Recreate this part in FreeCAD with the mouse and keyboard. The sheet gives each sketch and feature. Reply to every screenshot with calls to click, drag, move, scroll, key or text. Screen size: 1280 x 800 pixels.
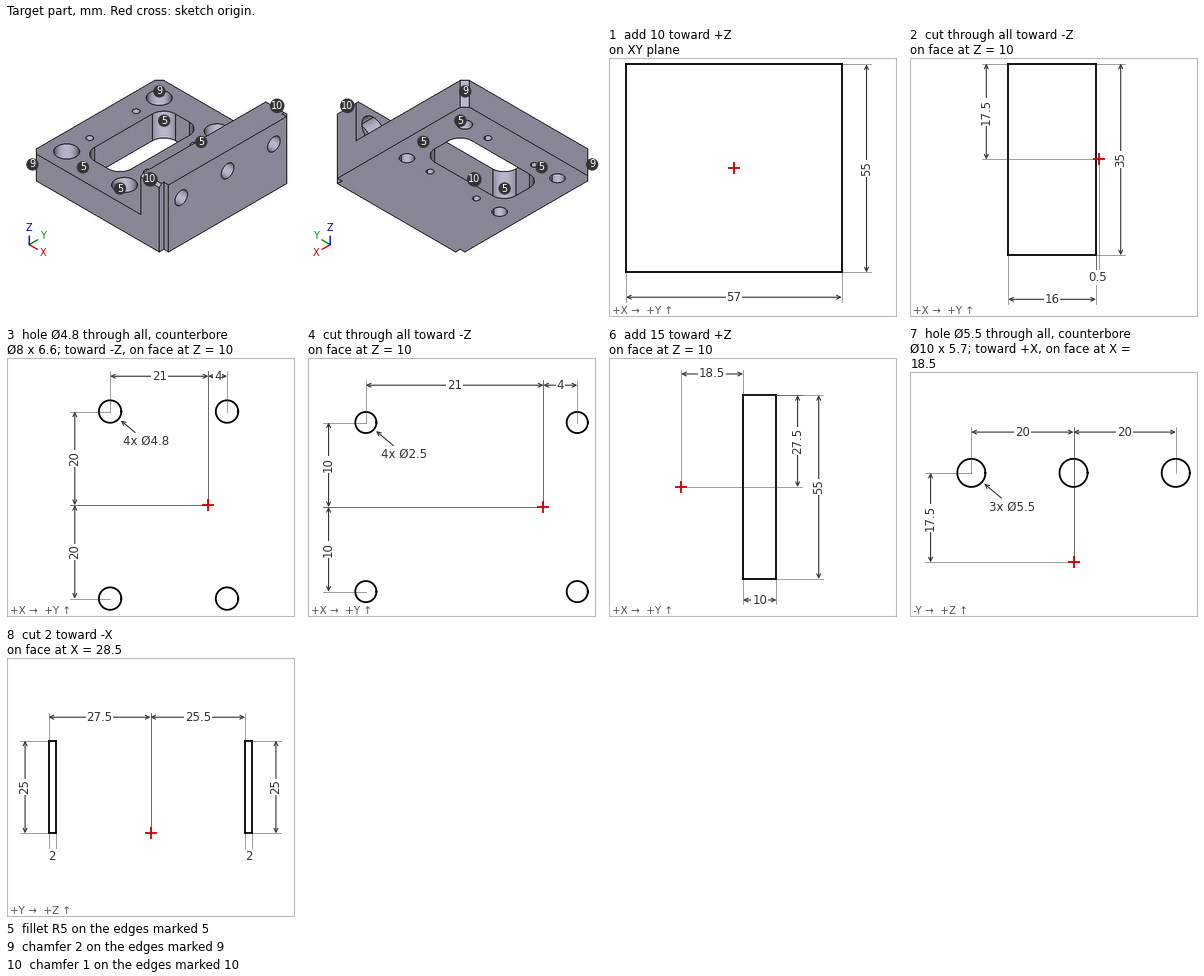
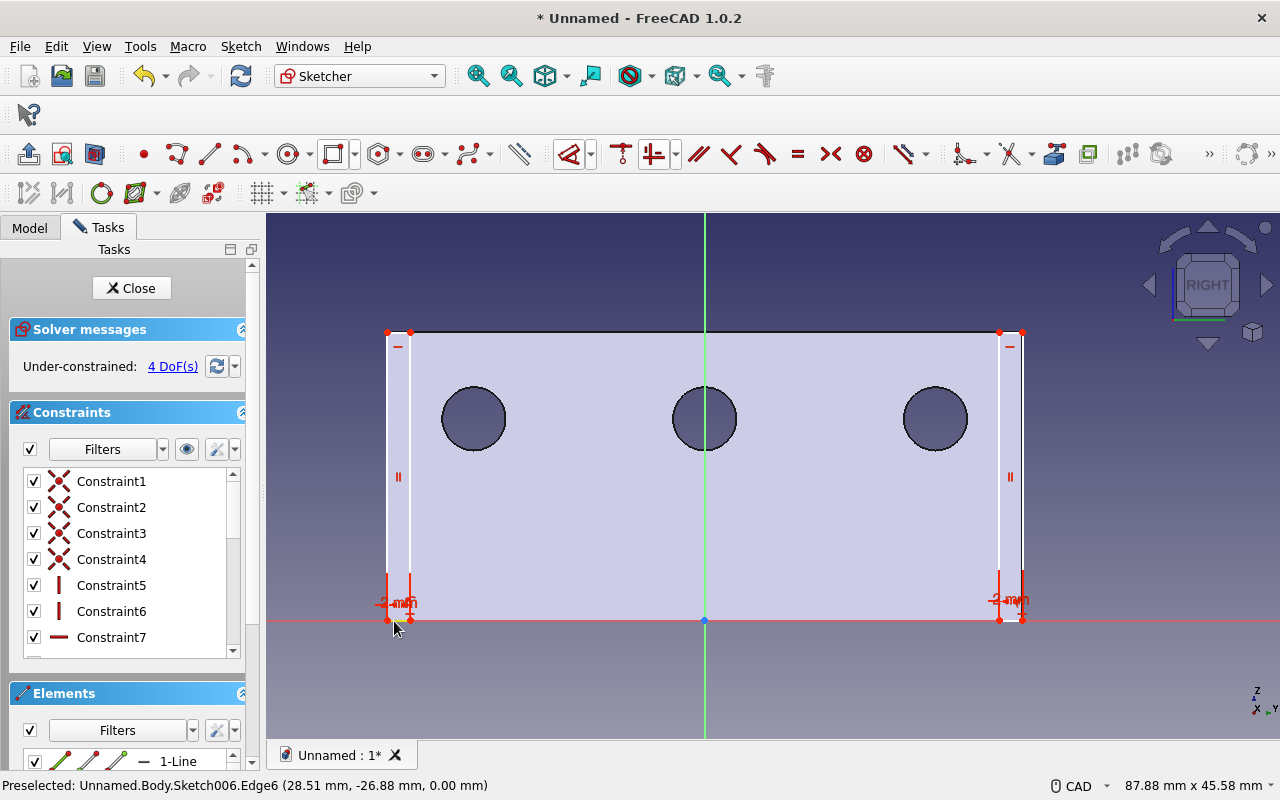
click(999, 419)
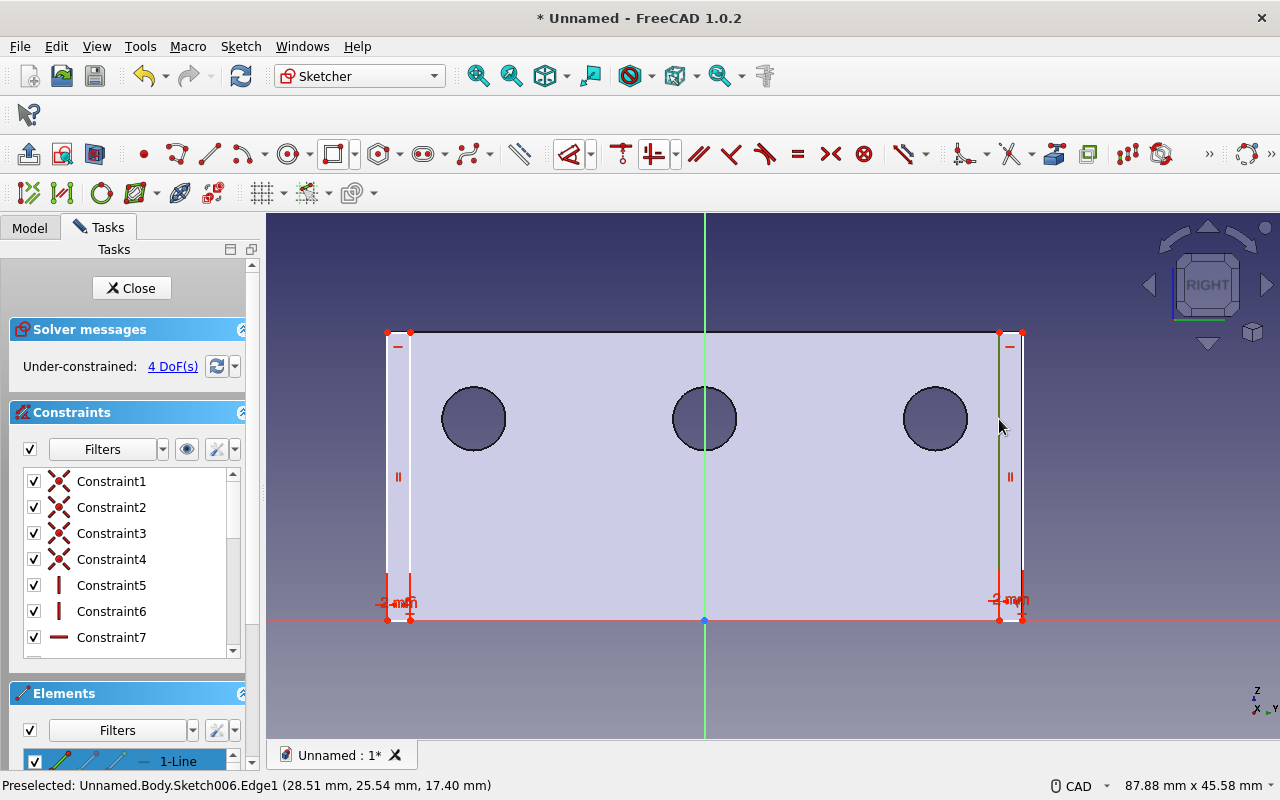
click(590, 154)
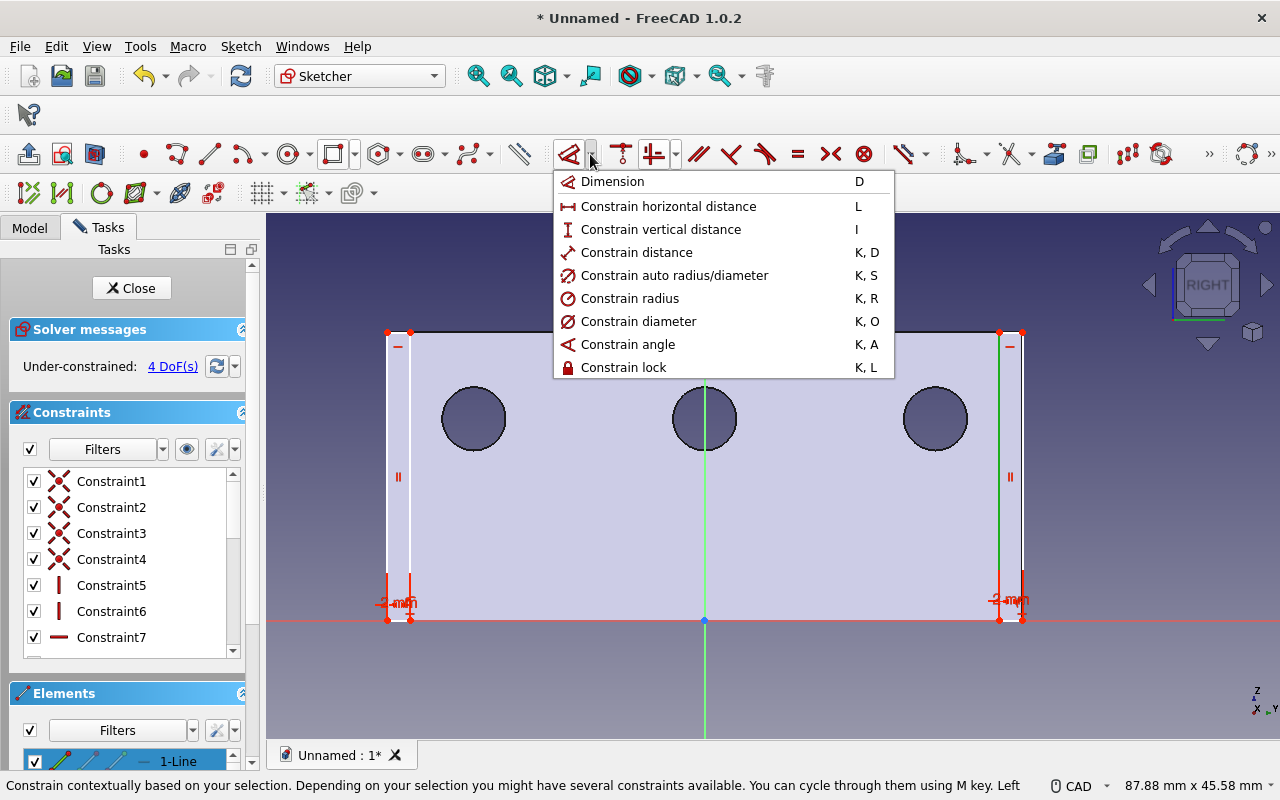
click(724, 230)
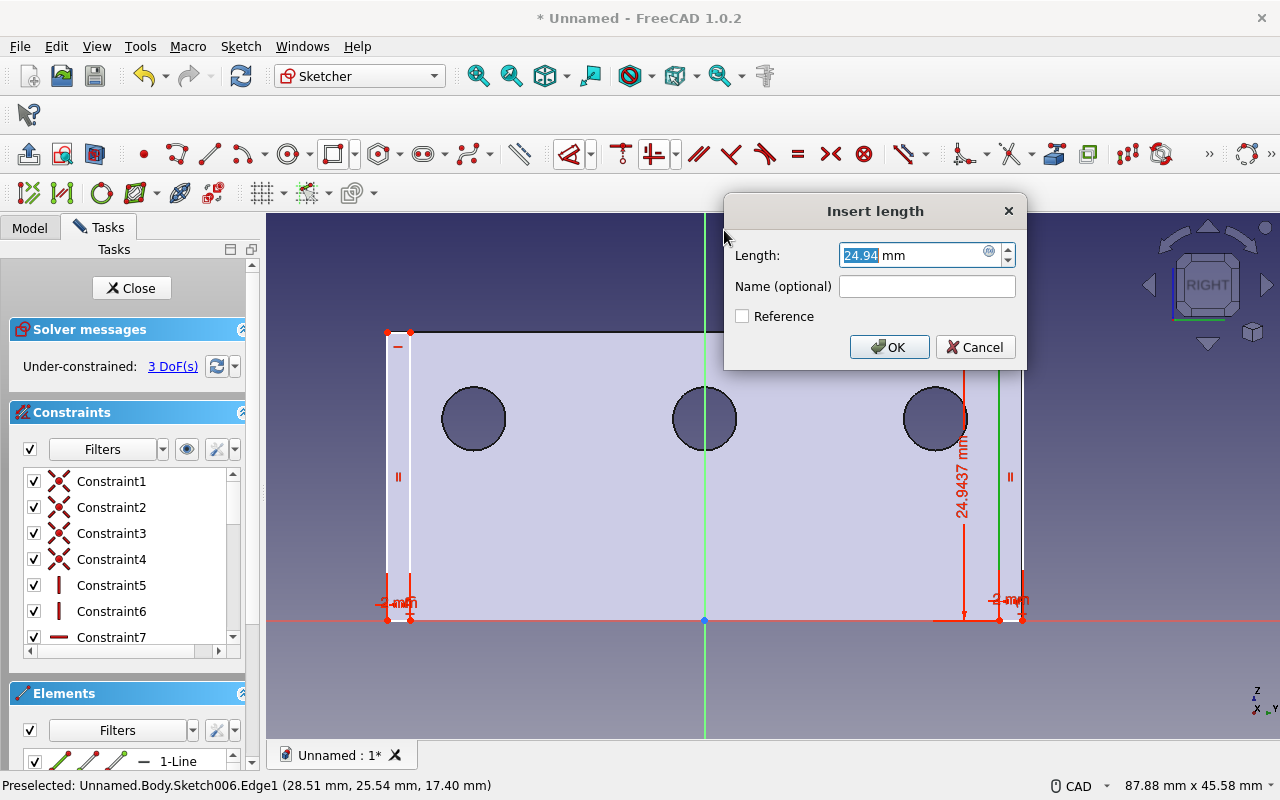
text(25)
key(Return)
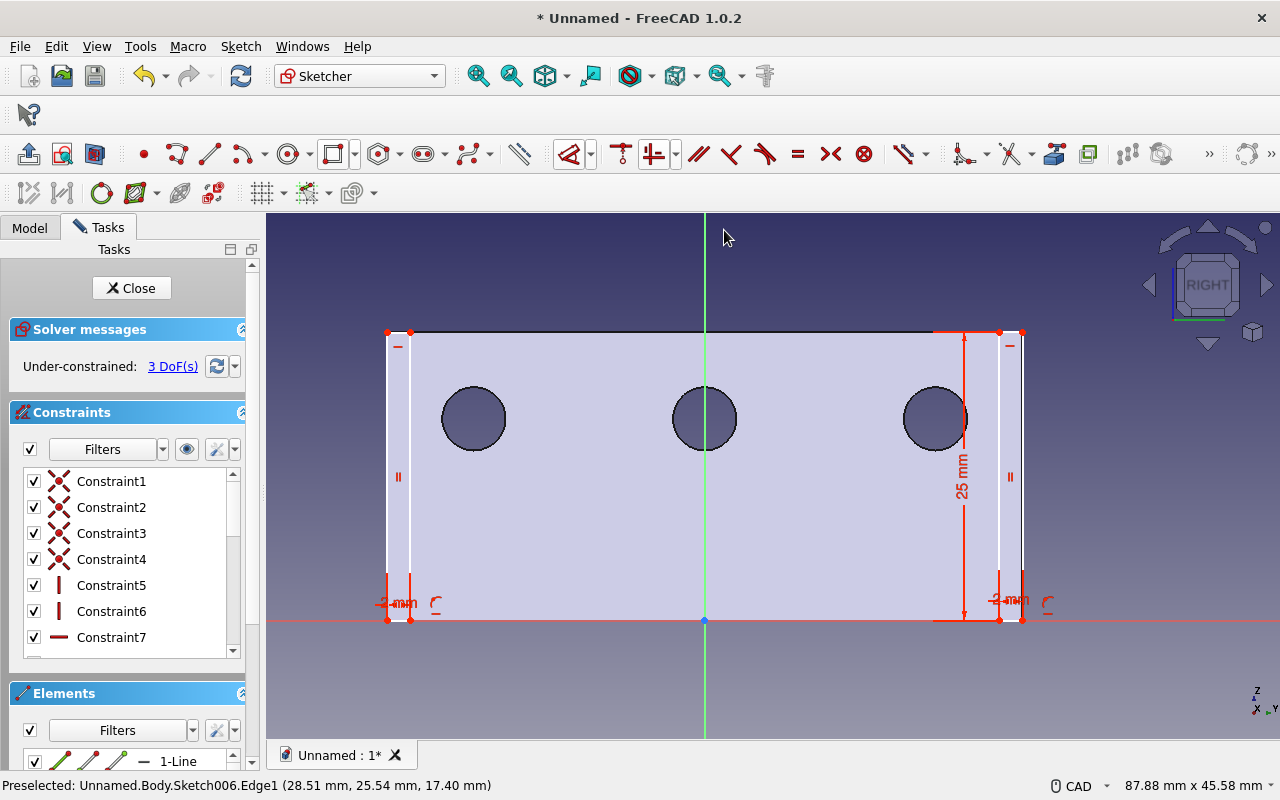
click(387, 419)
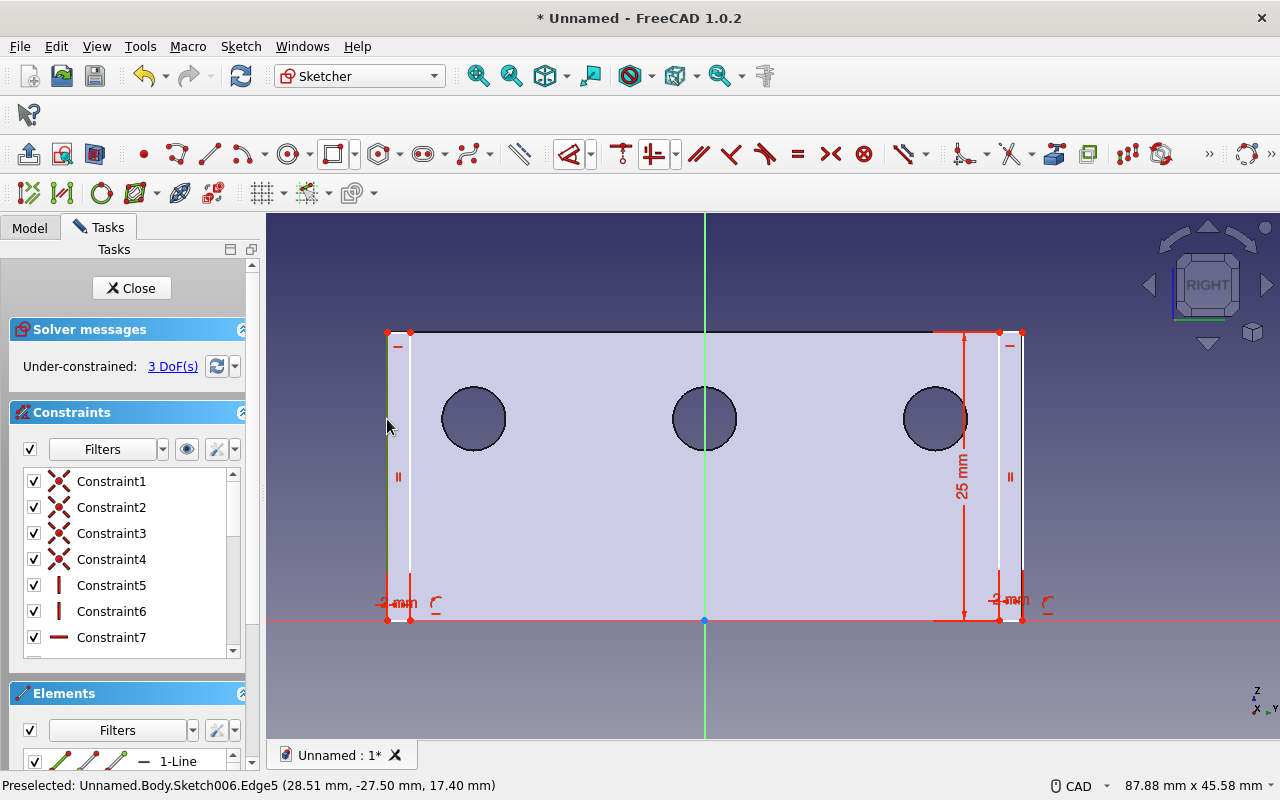
key(i)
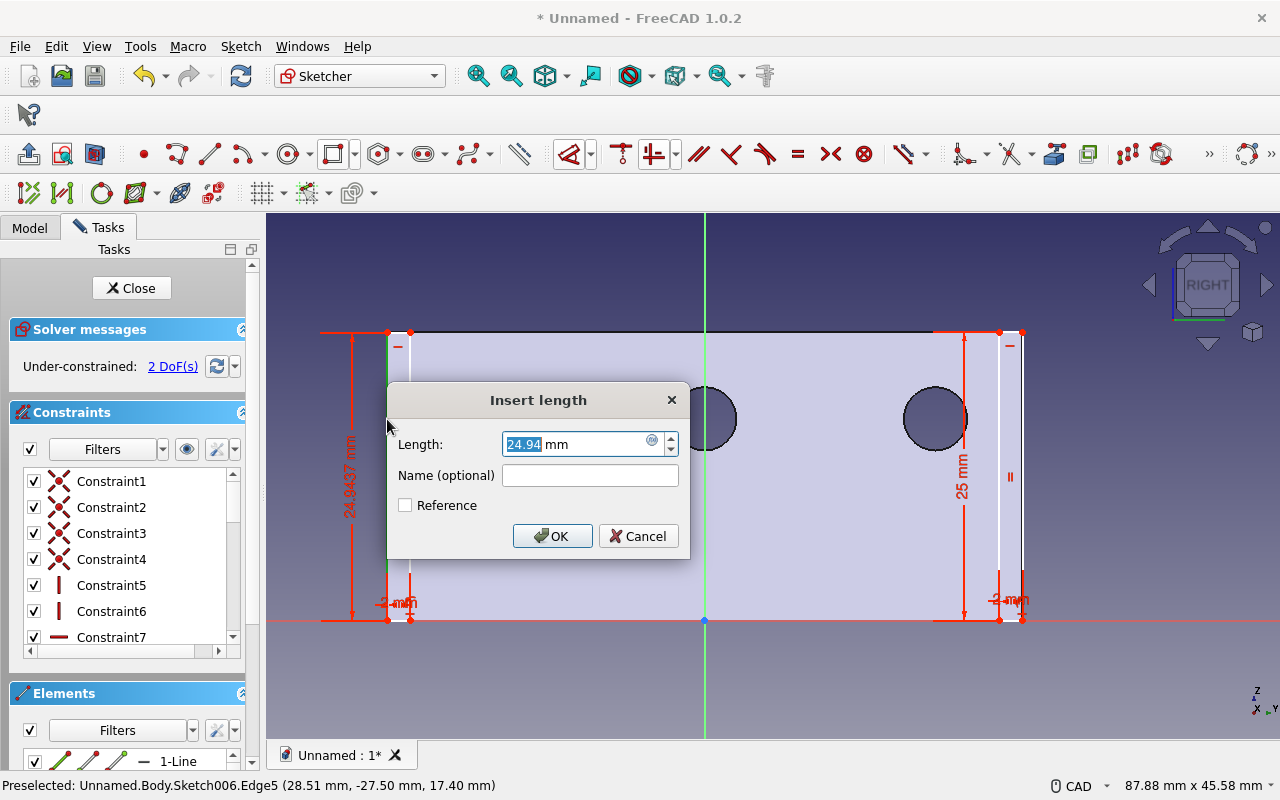
text(25)
key(Return)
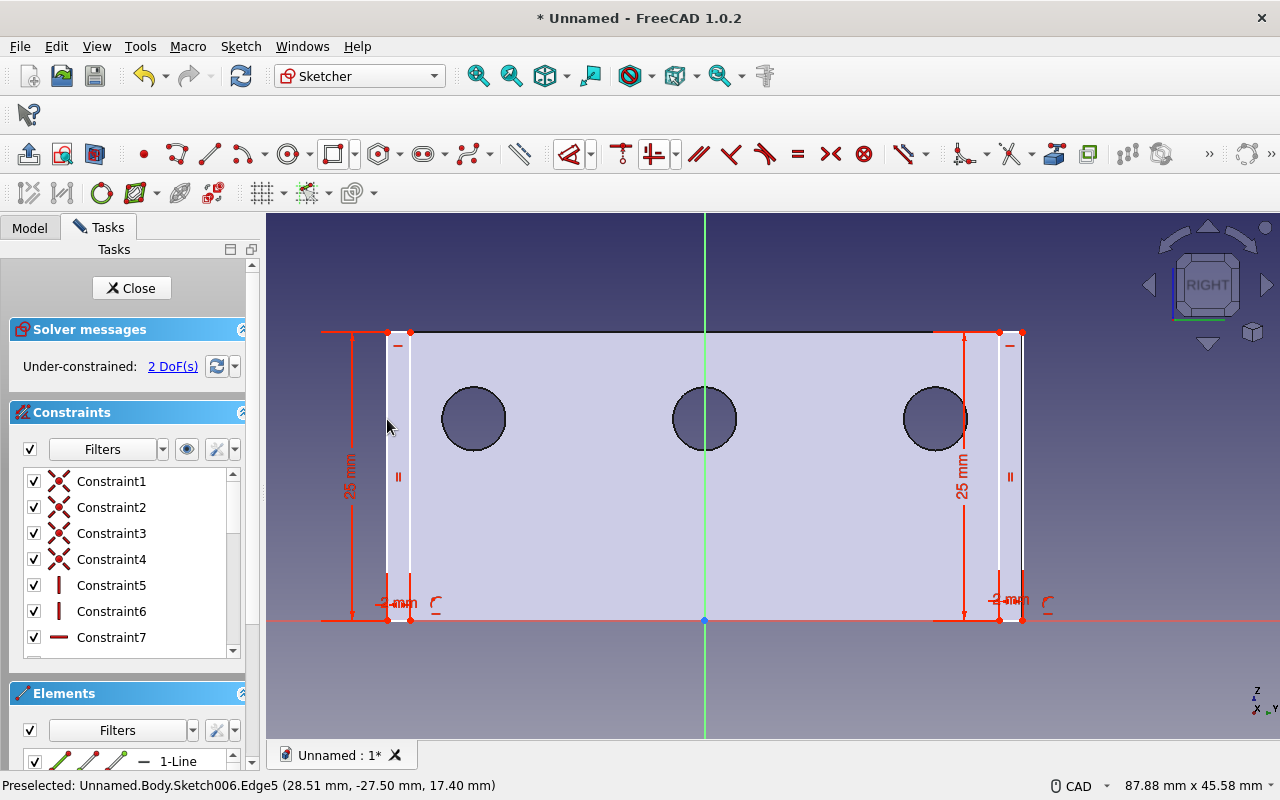
click(999, 332)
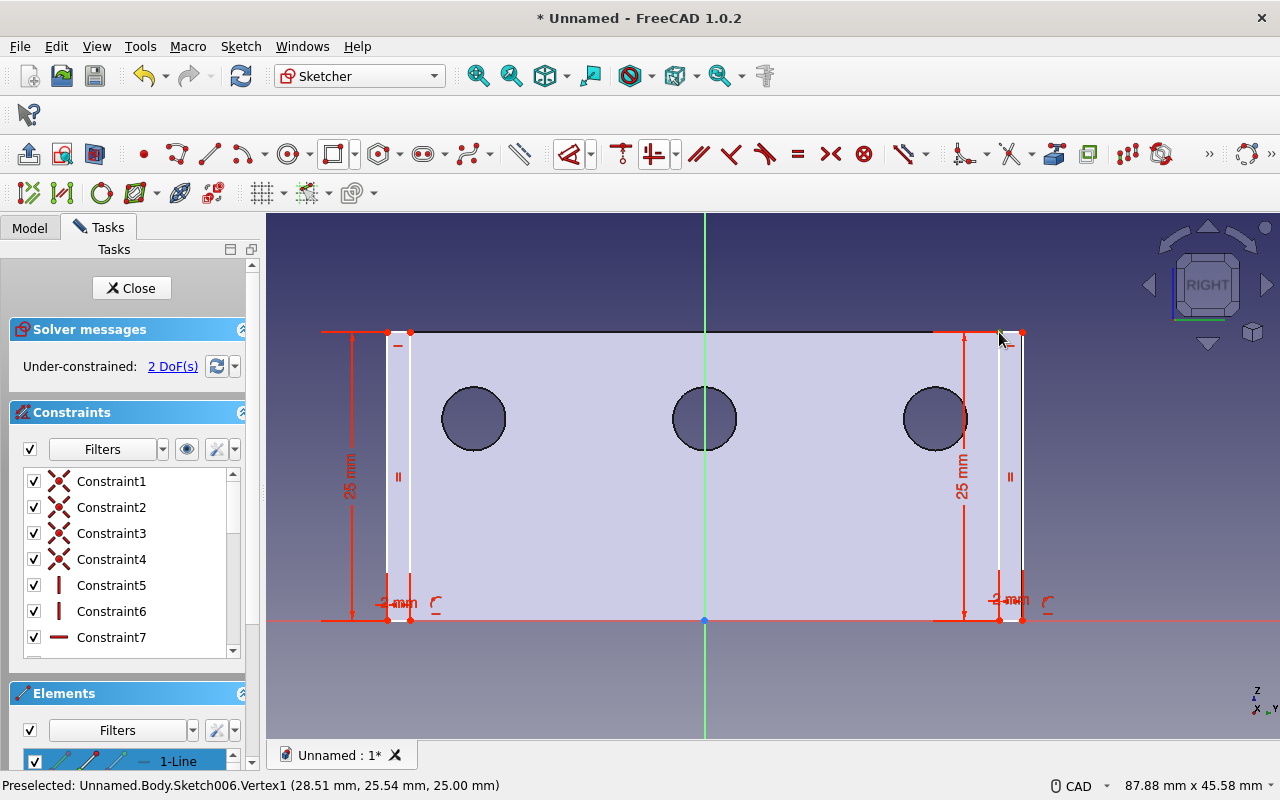
click(590, 154)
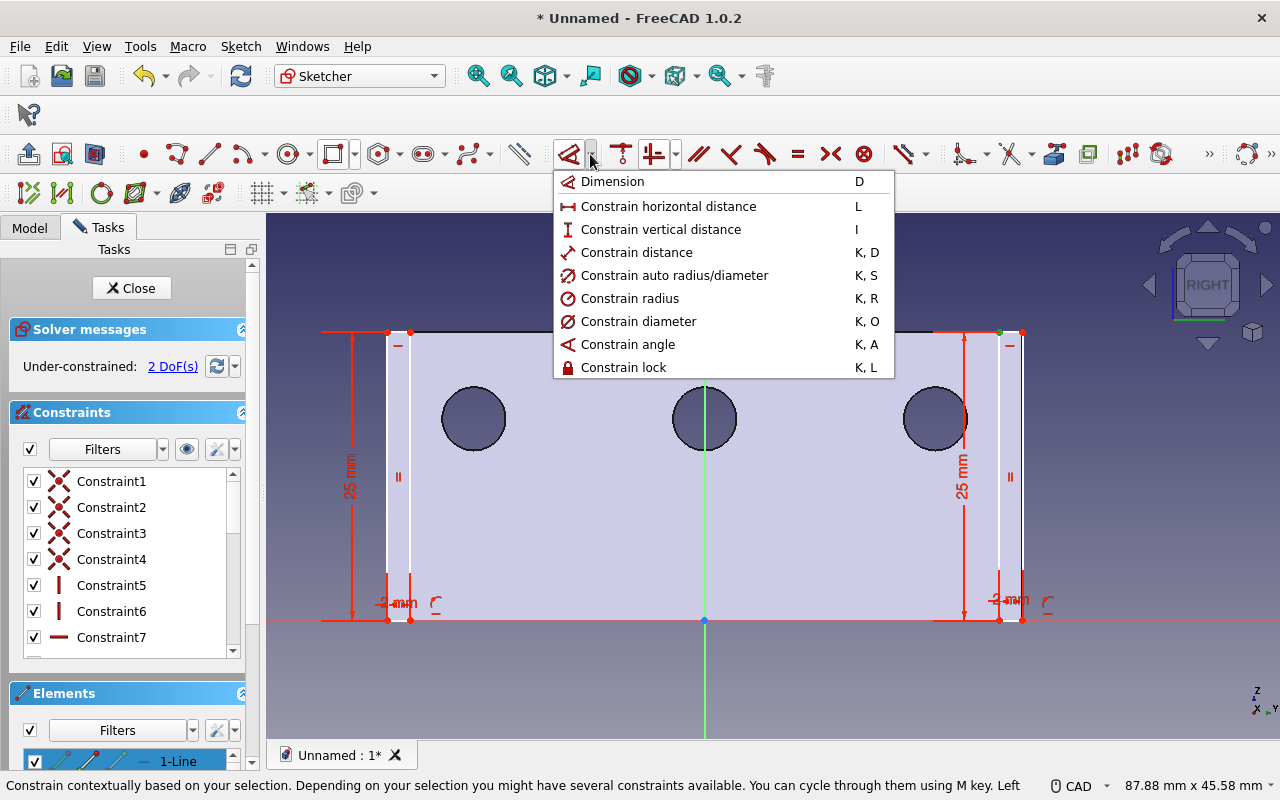
click(724, 206)